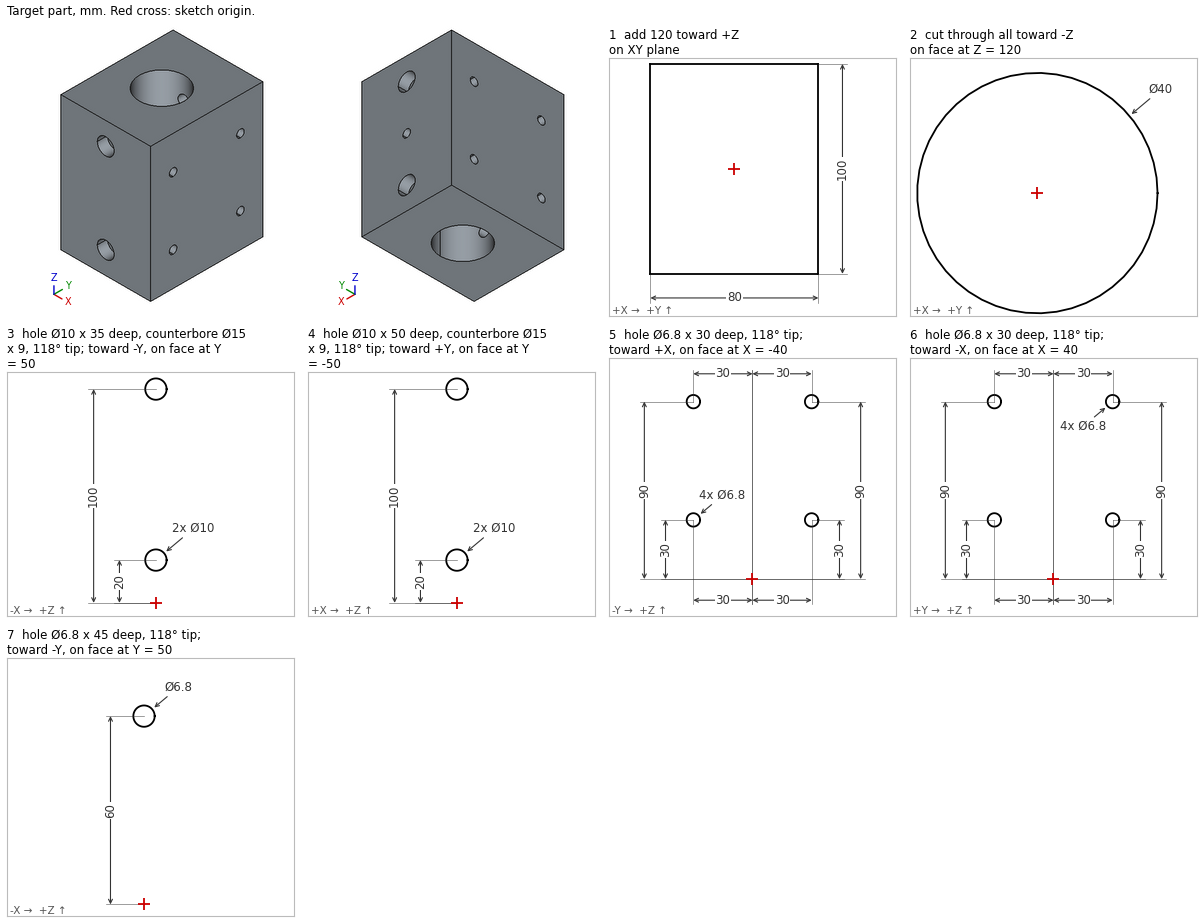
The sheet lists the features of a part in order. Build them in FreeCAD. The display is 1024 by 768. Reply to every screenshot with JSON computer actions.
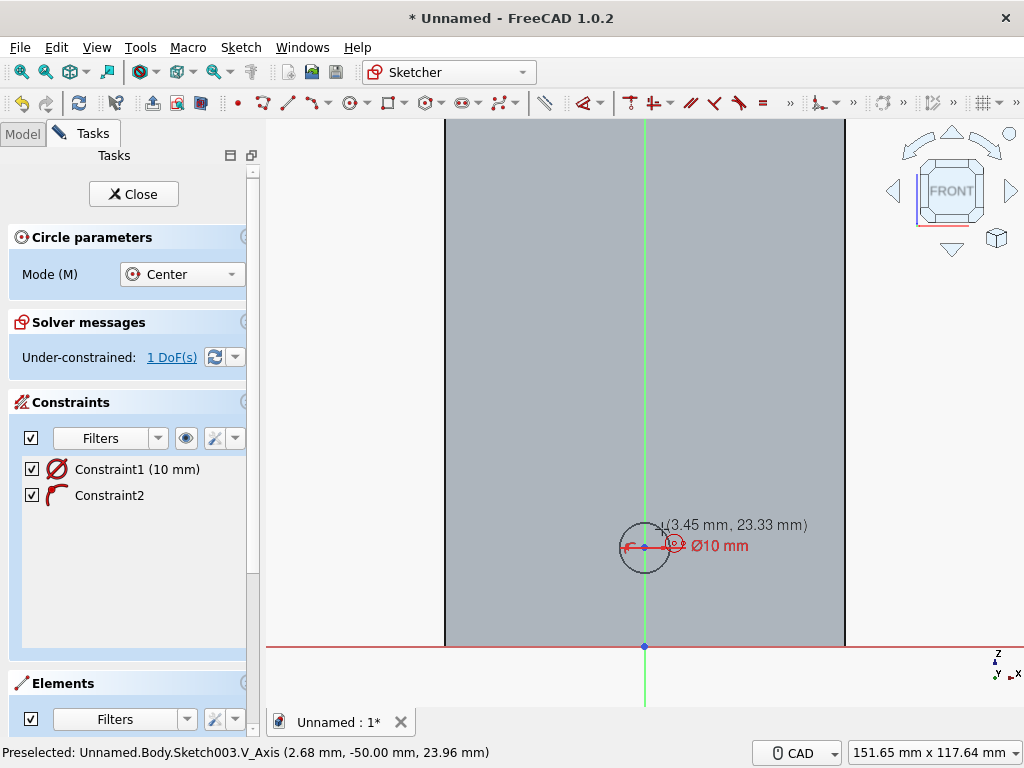
{"action": "scroll", "coordinate": [438, 472], "scroll_direction": "down", "scroll_amount": 2}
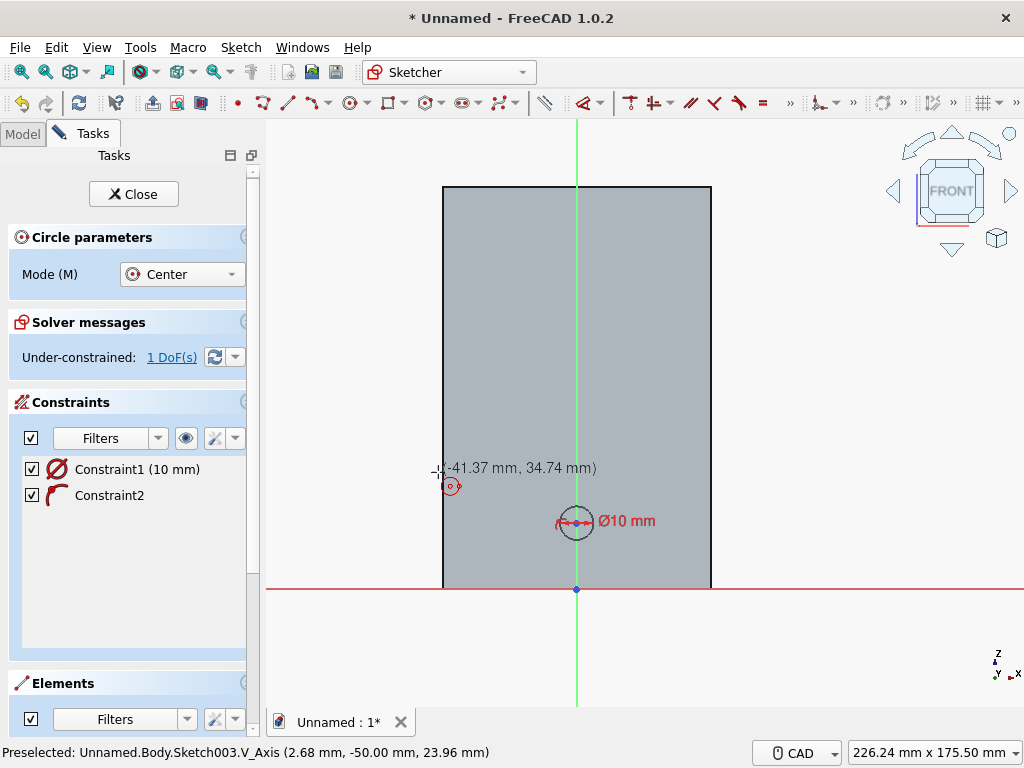
{"action": "scroll", "coordinate": [577, 254], "scroll_direction": "up", "scroll_amount": 2}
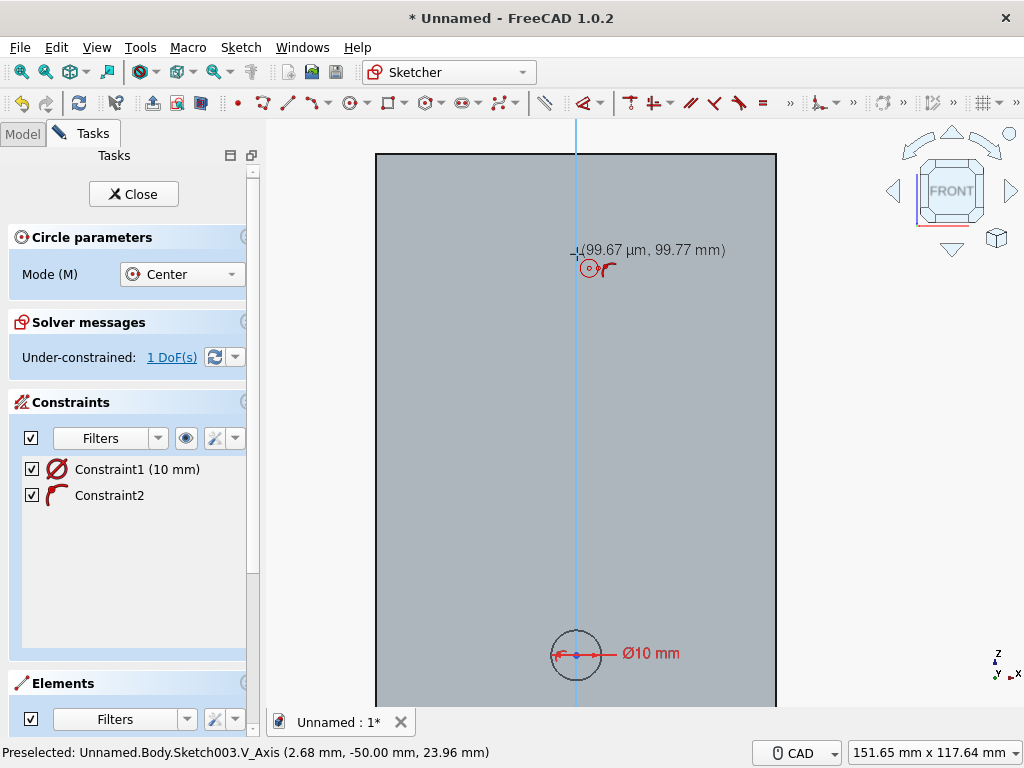
{"action": "left_click", "coordinate": [576, 254]}
{"action": "mouse_move", "coordinate": [594, 237]}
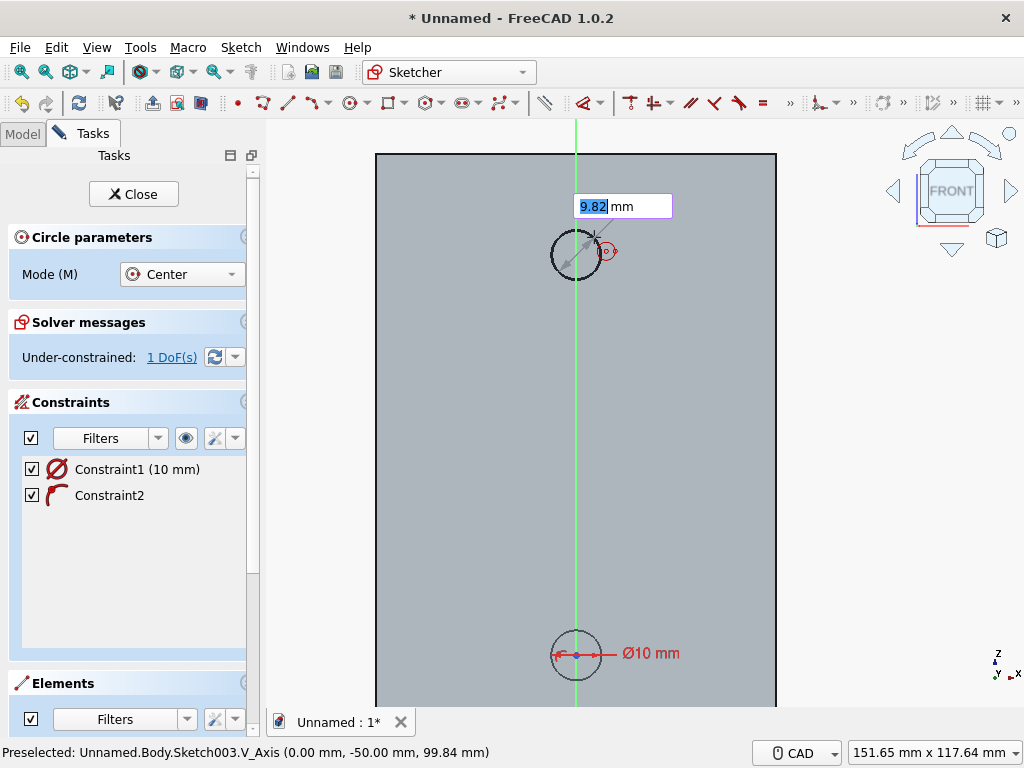
{"action": "type", "text": "10"}
{"action": "key", "text": "Return"}
{"action": "key", "text": "Escape"}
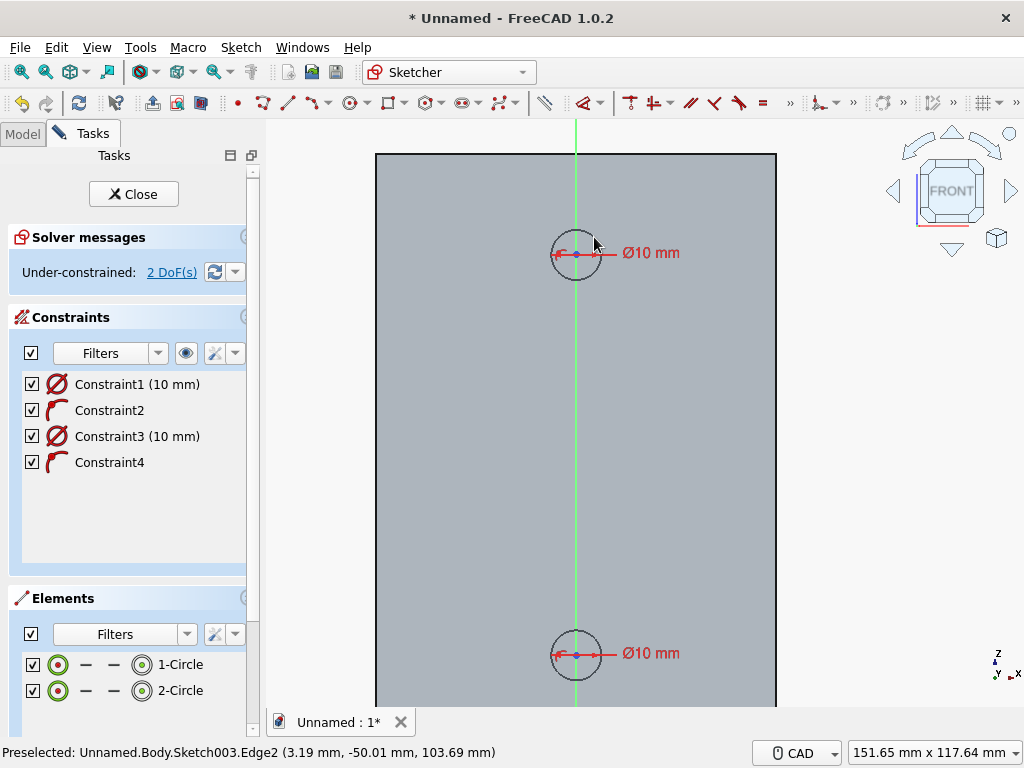
{"action": "left_click", "coordinate": [584, 104]}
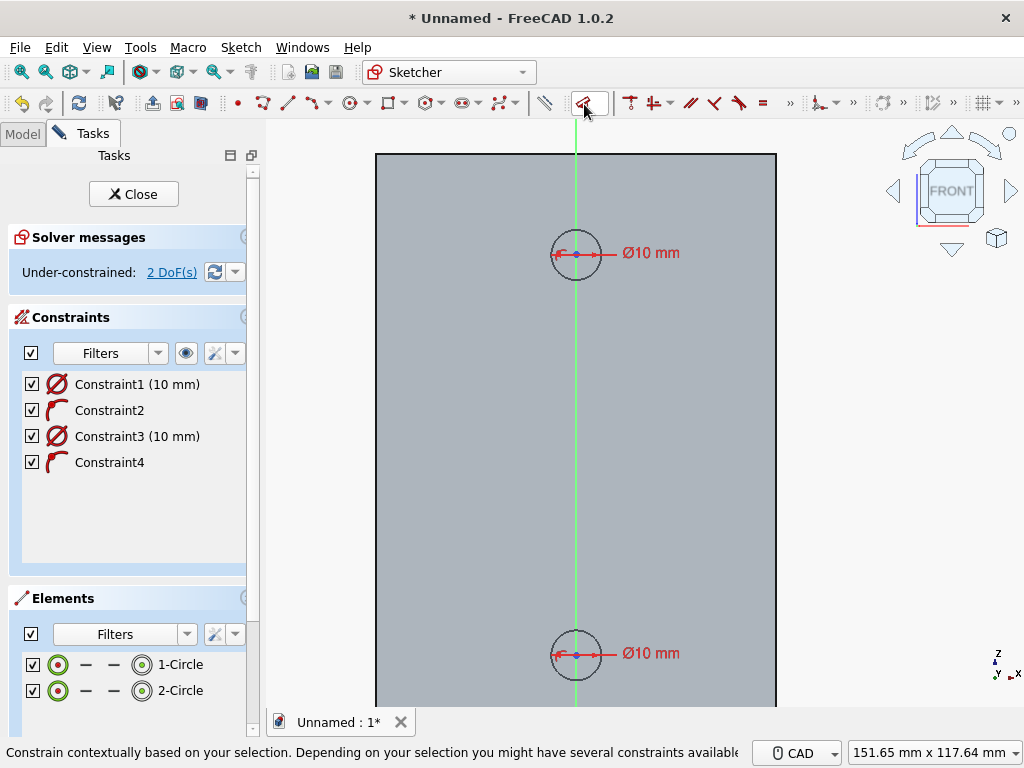
{"action": "left_click", "coordinate": [576, 655]}
{"action": "left_click", "coordinate": [610, 673]}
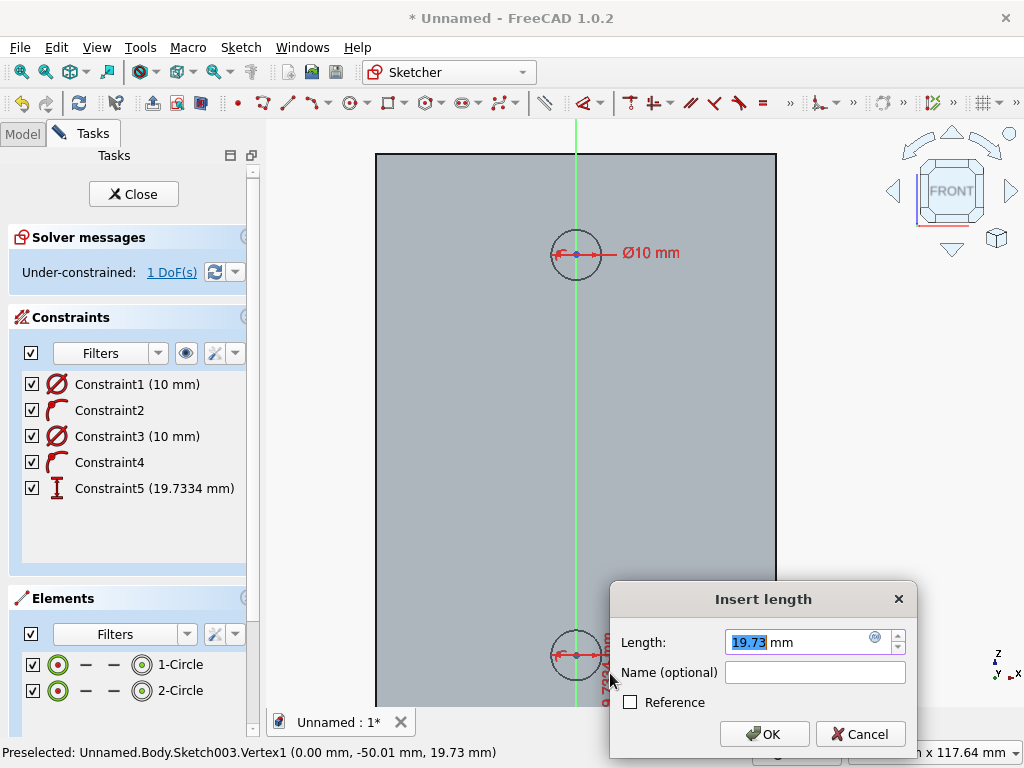
{"action": "type", "text": "20"}
{"action": "key", "text": "Return"}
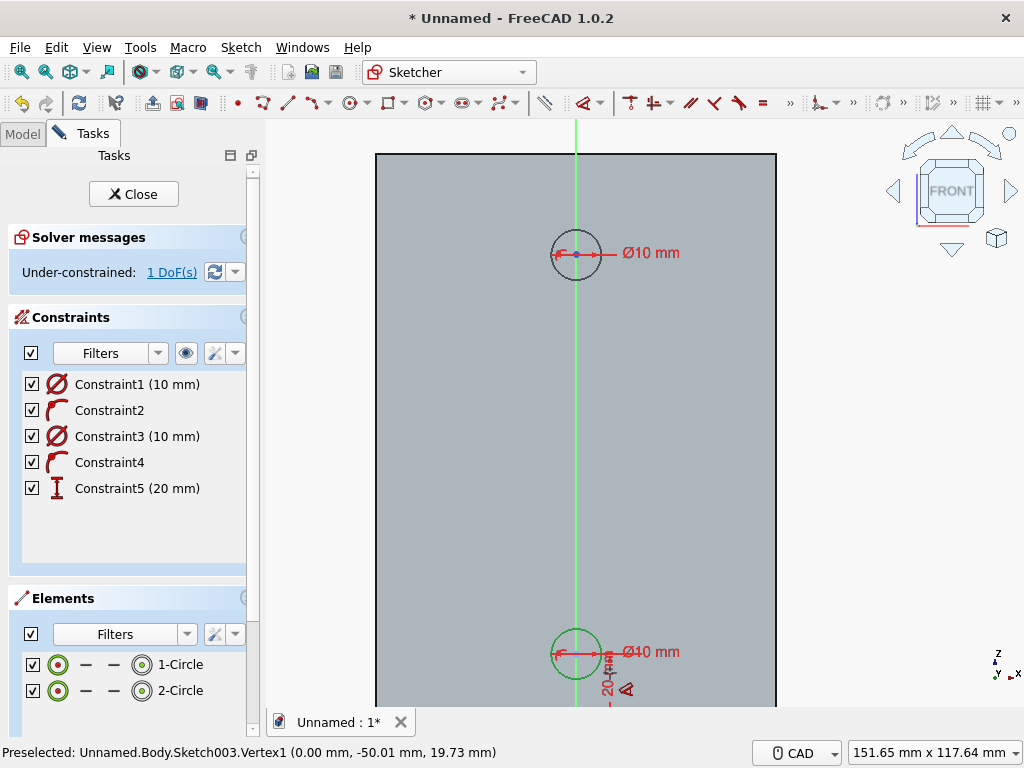
{"action": "left_click", "coordinate": [576, 255]}
{"action": "left_click", "coordinate": [610, 467]}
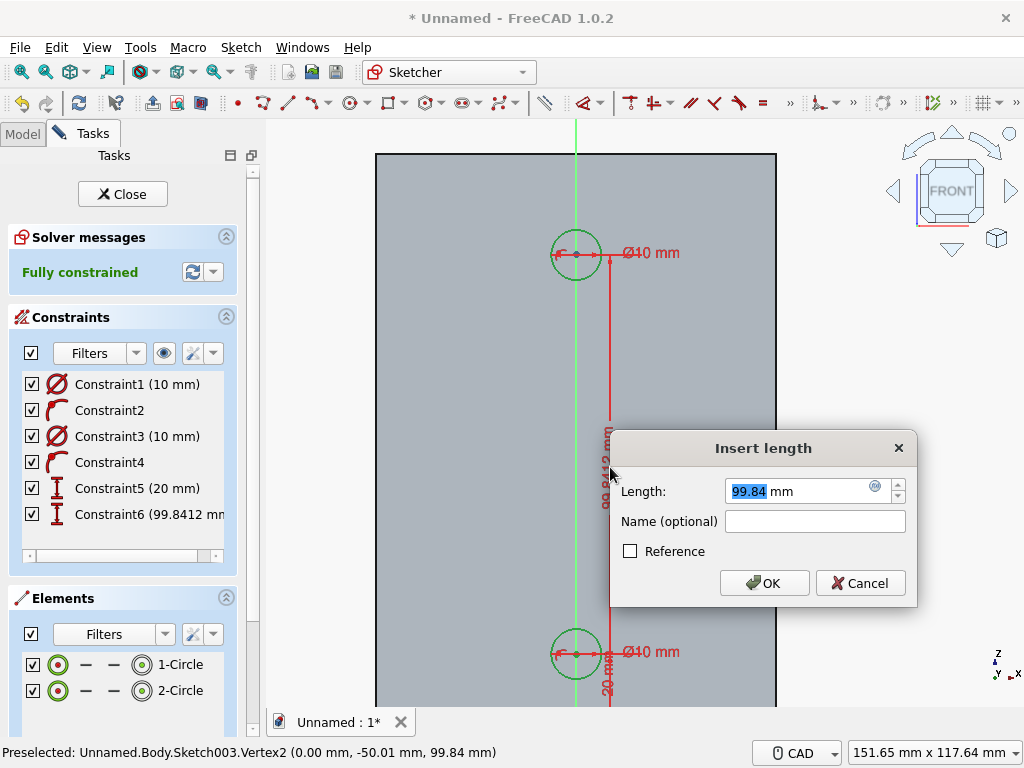
{"action": "type", "text": "100"}
{"action": "key", "text": "Return"}
{"action": "key", "text": "Escape"}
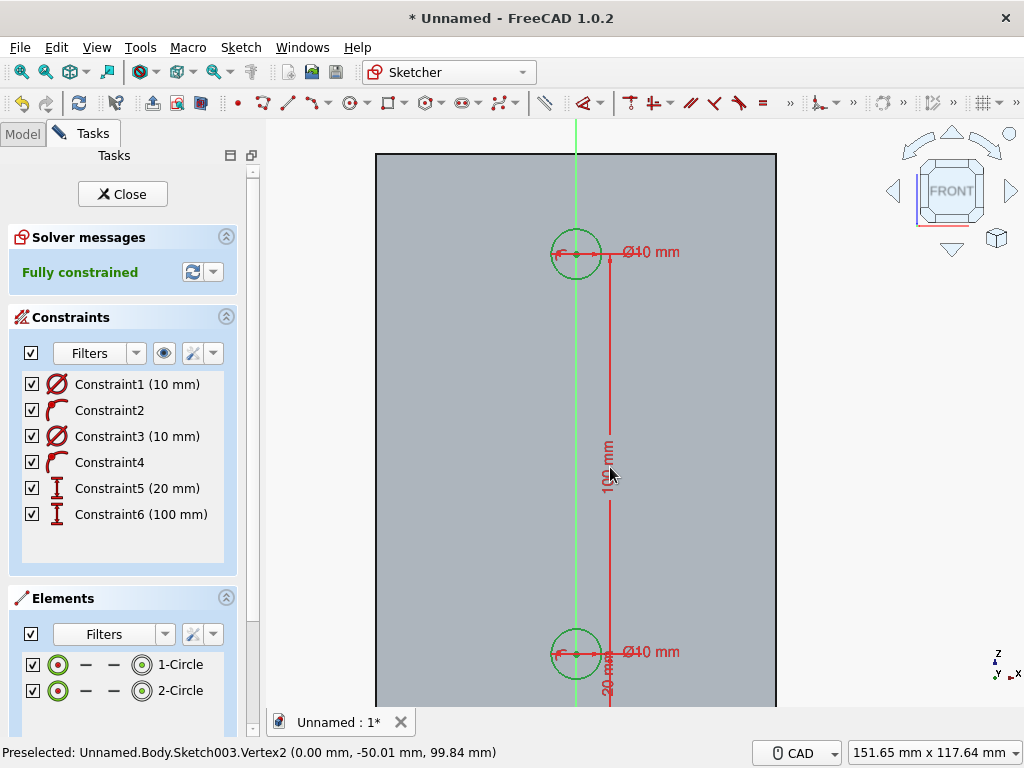
{"action": "left_click", "coordinate": [123, 194]}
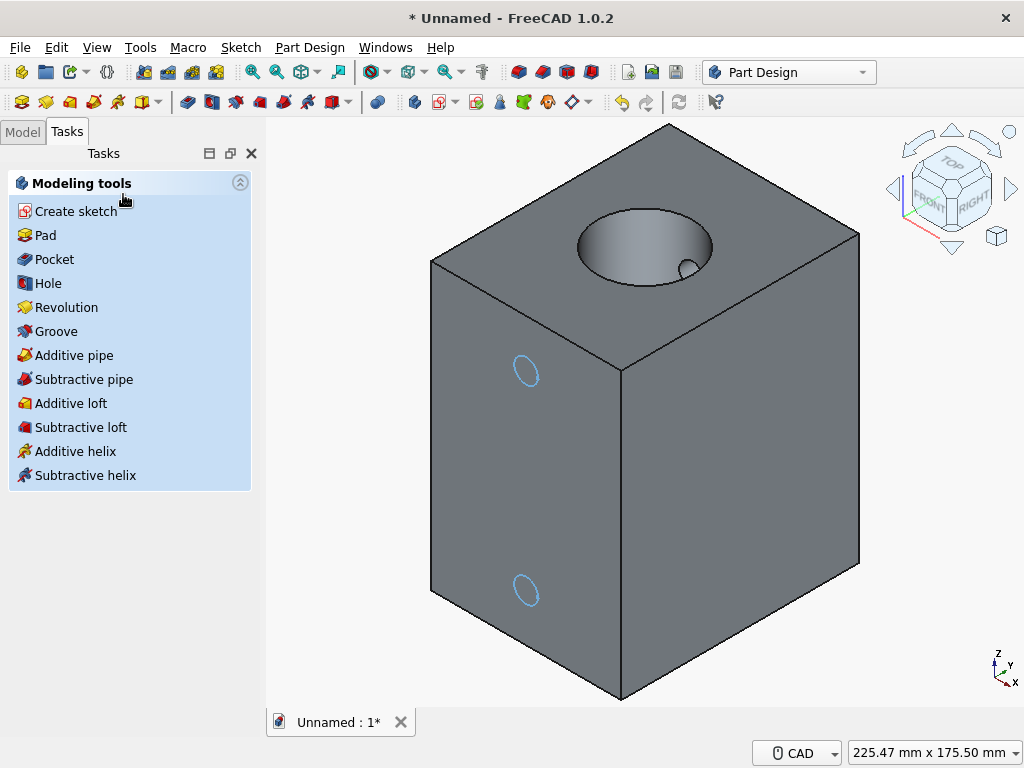
{"action": "left_click", "coordinate": [212, 102]}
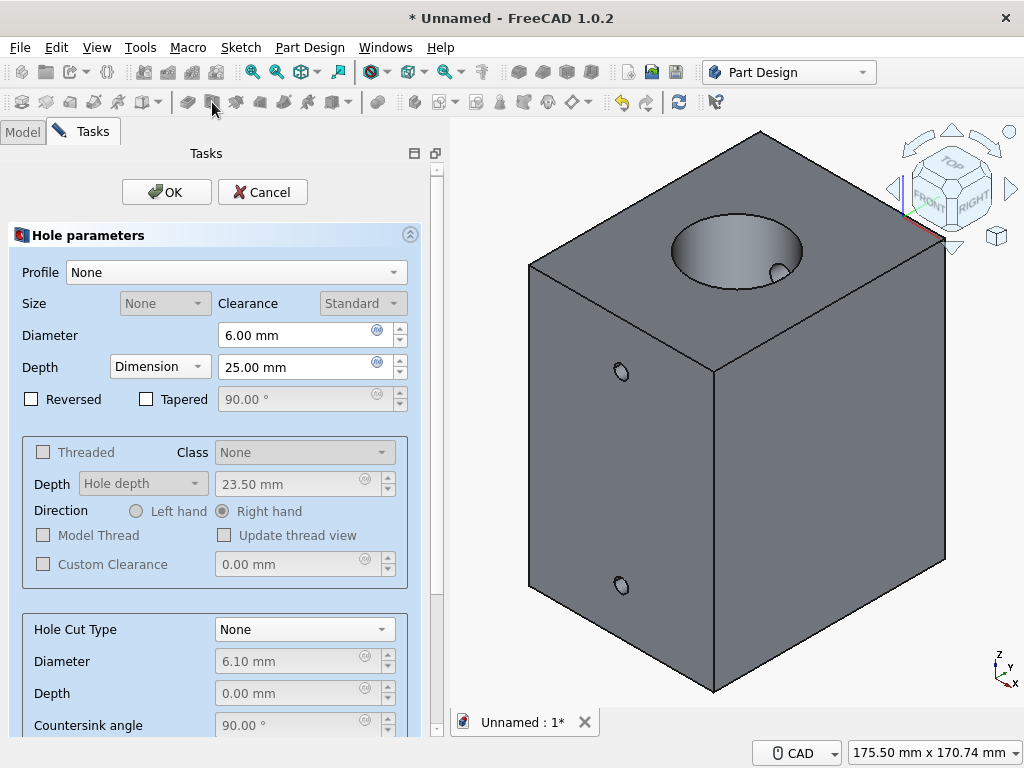
{"action": "triple_click", "coordinate": [305, 335]}